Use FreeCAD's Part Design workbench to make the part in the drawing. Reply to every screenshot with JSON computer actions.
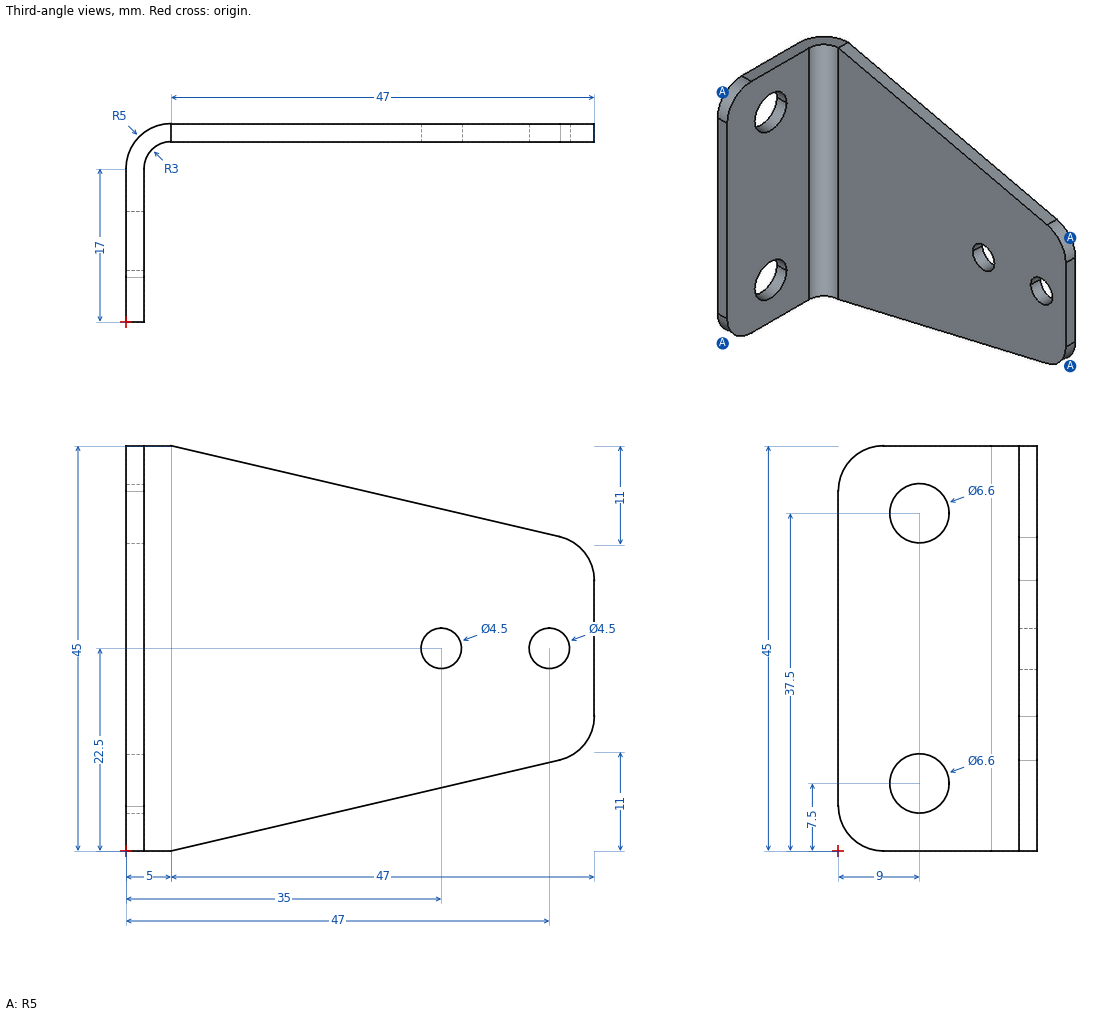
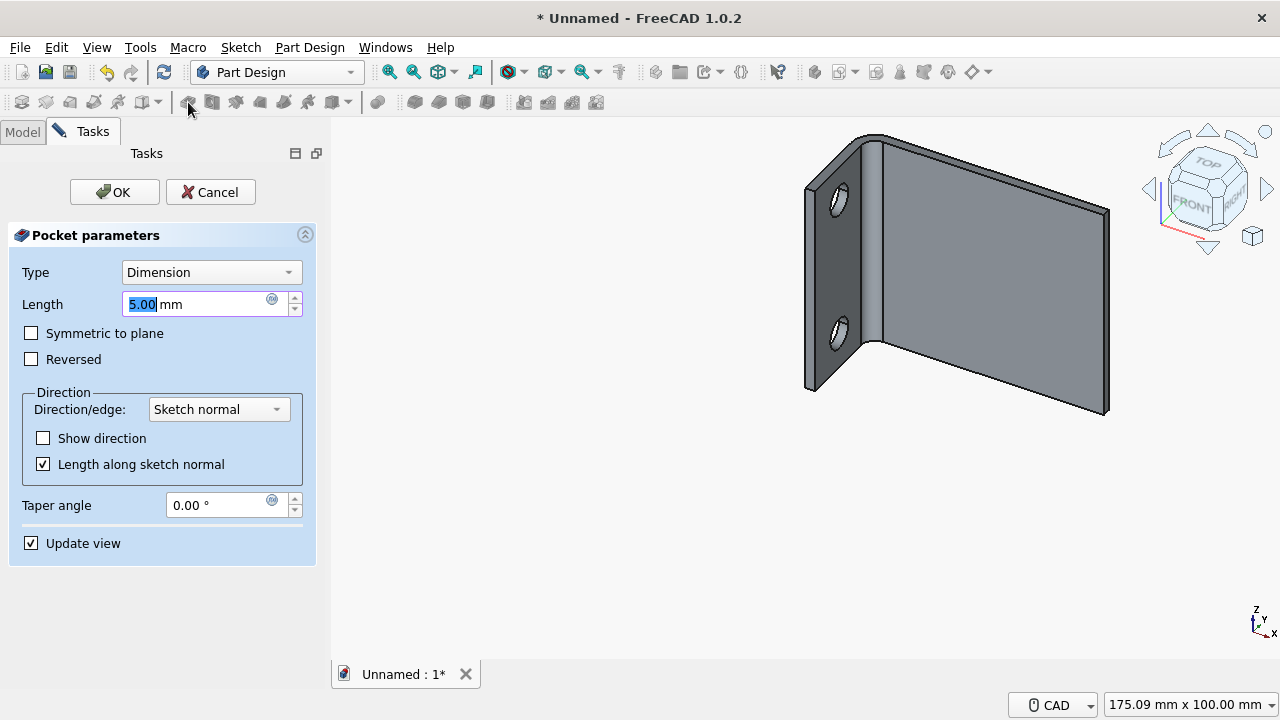
{"action": "left_click", "coordinate": [212, 272]}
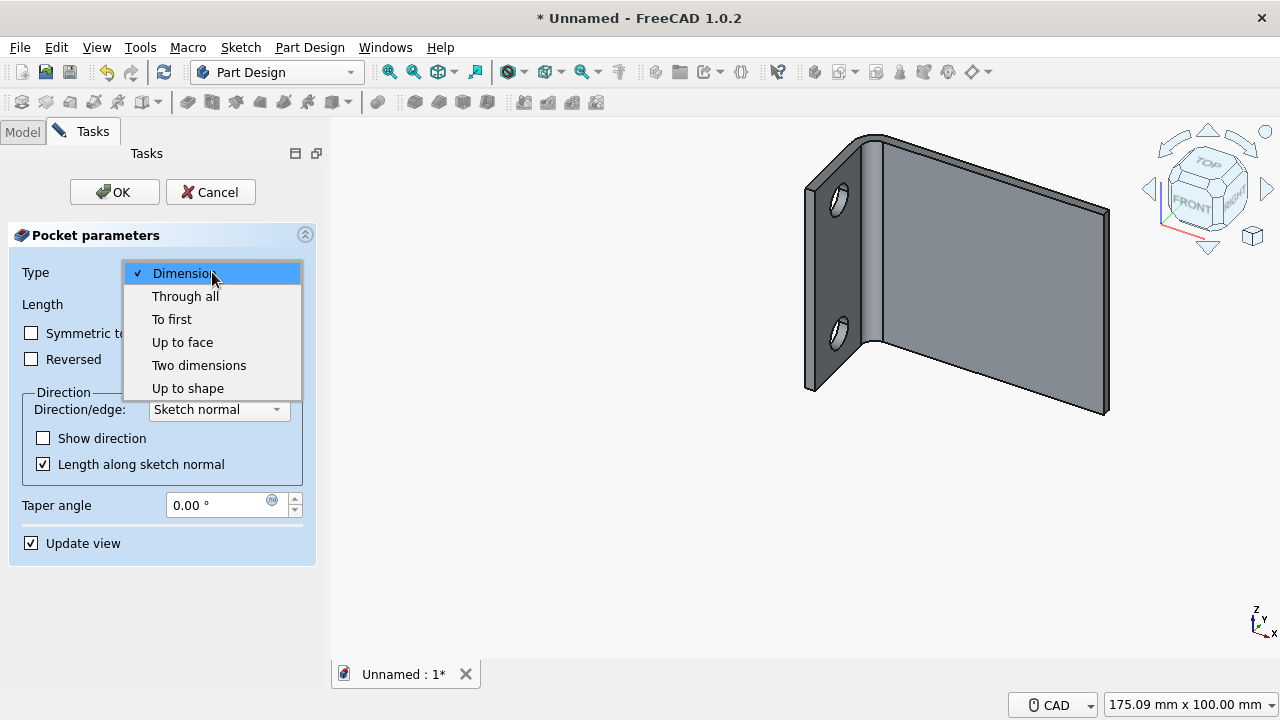
{"action": "left_click", "coordinate": [212, 320]}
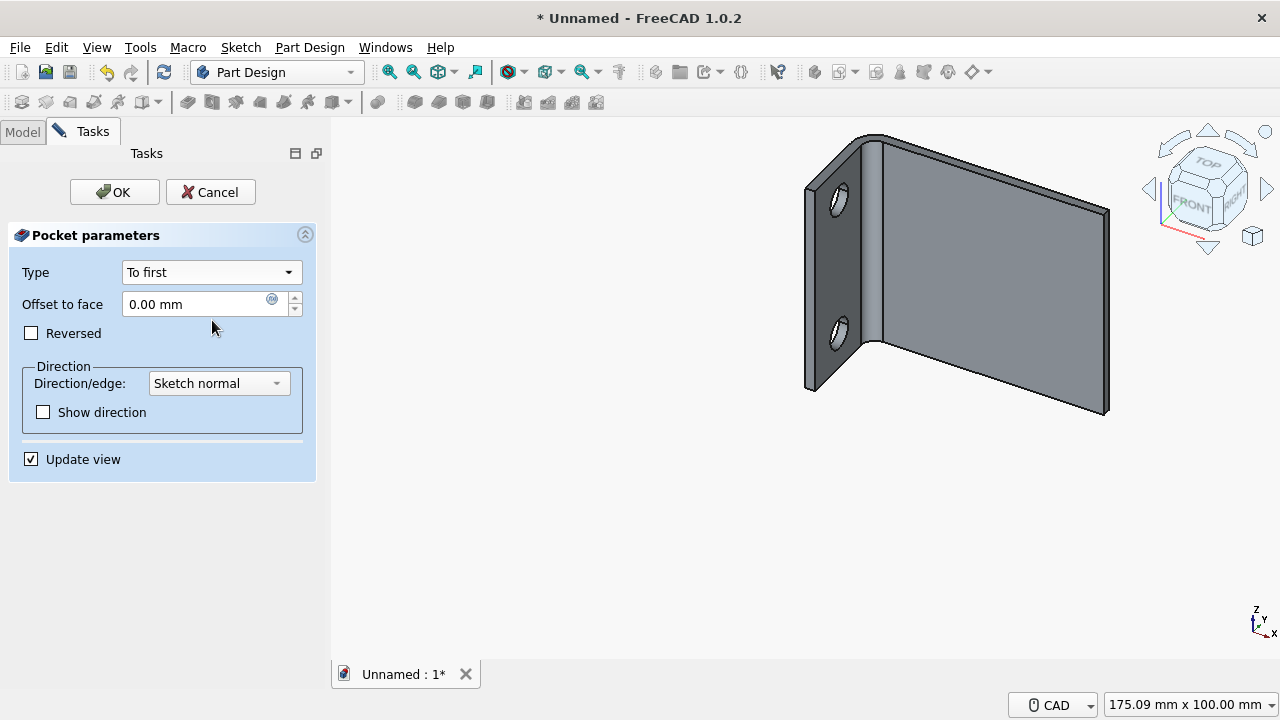
{"action": "left_click", "coordinate": [115, 192]}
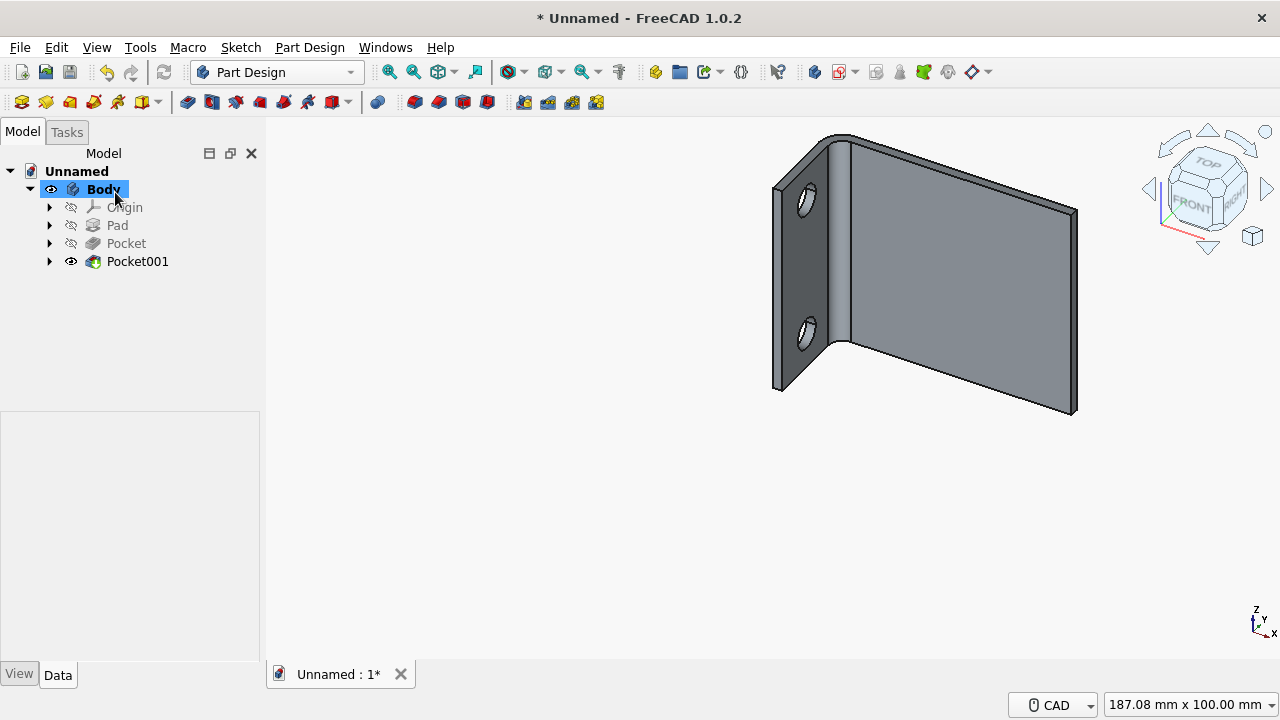
{"action": "key", "text": "4"}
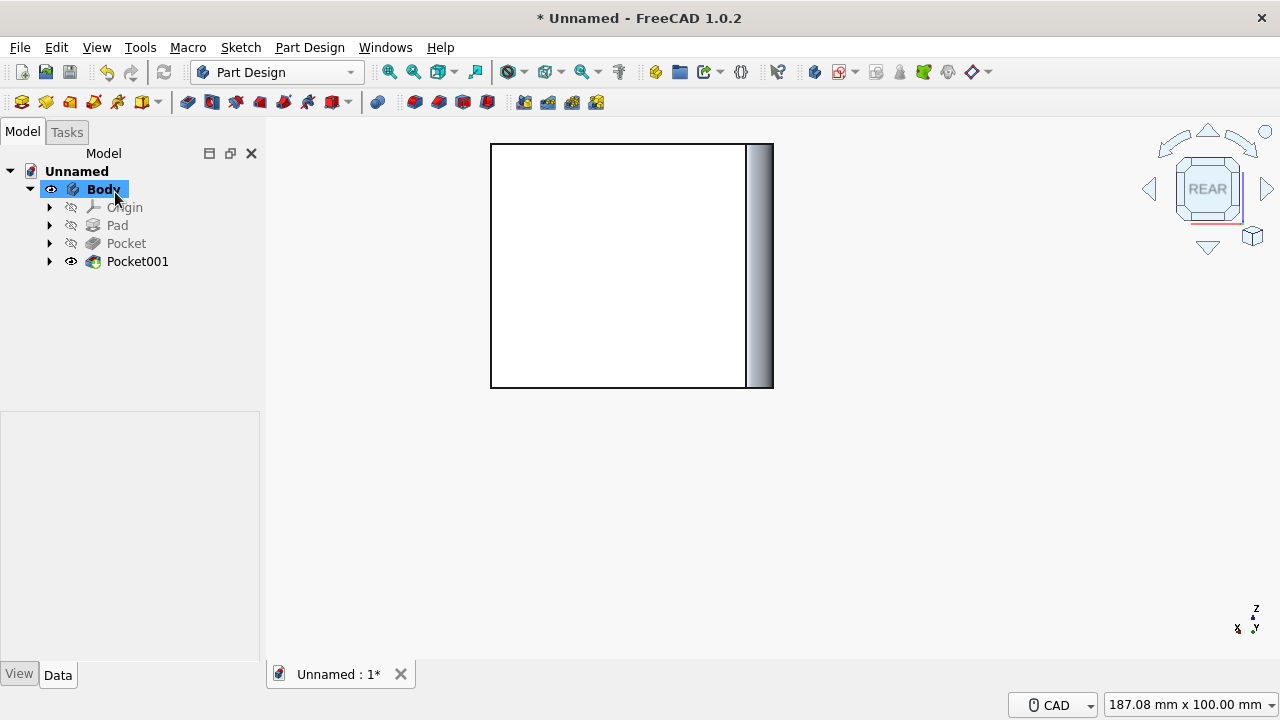
{"action": "left_click", "coordinate": [619, 265]}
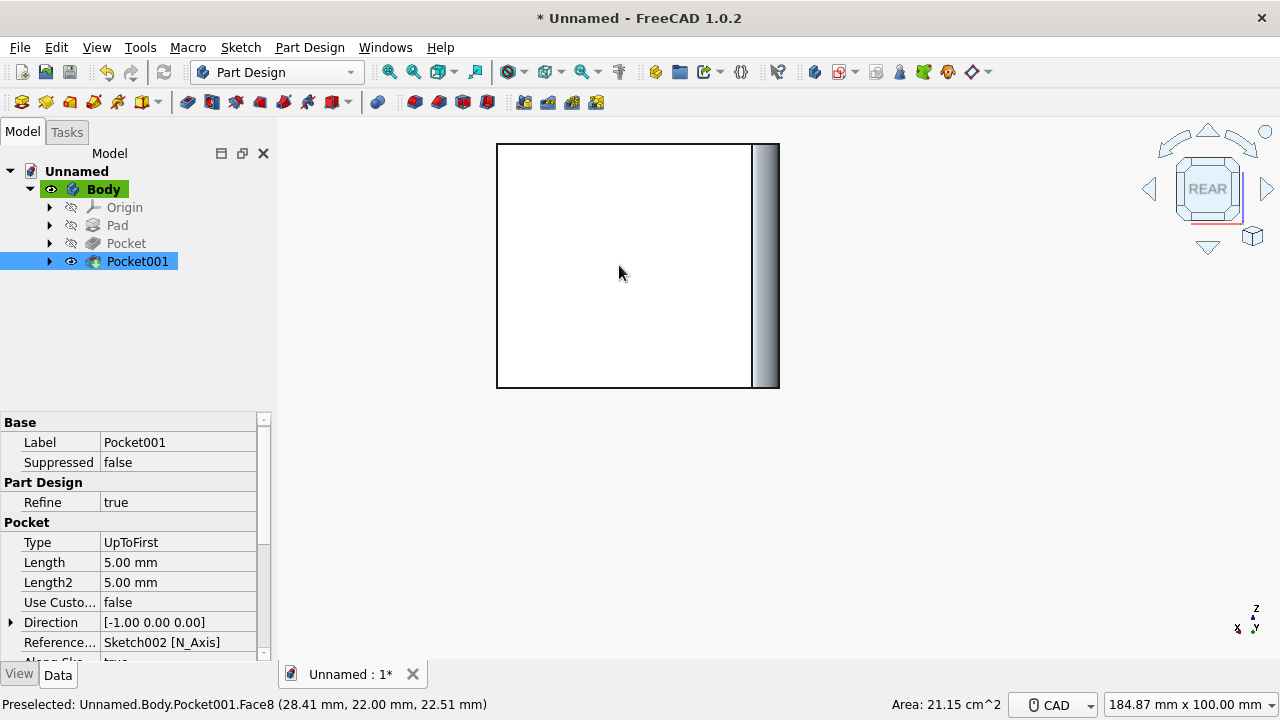
{"action": "left_click", "coordinate": [840, 72]}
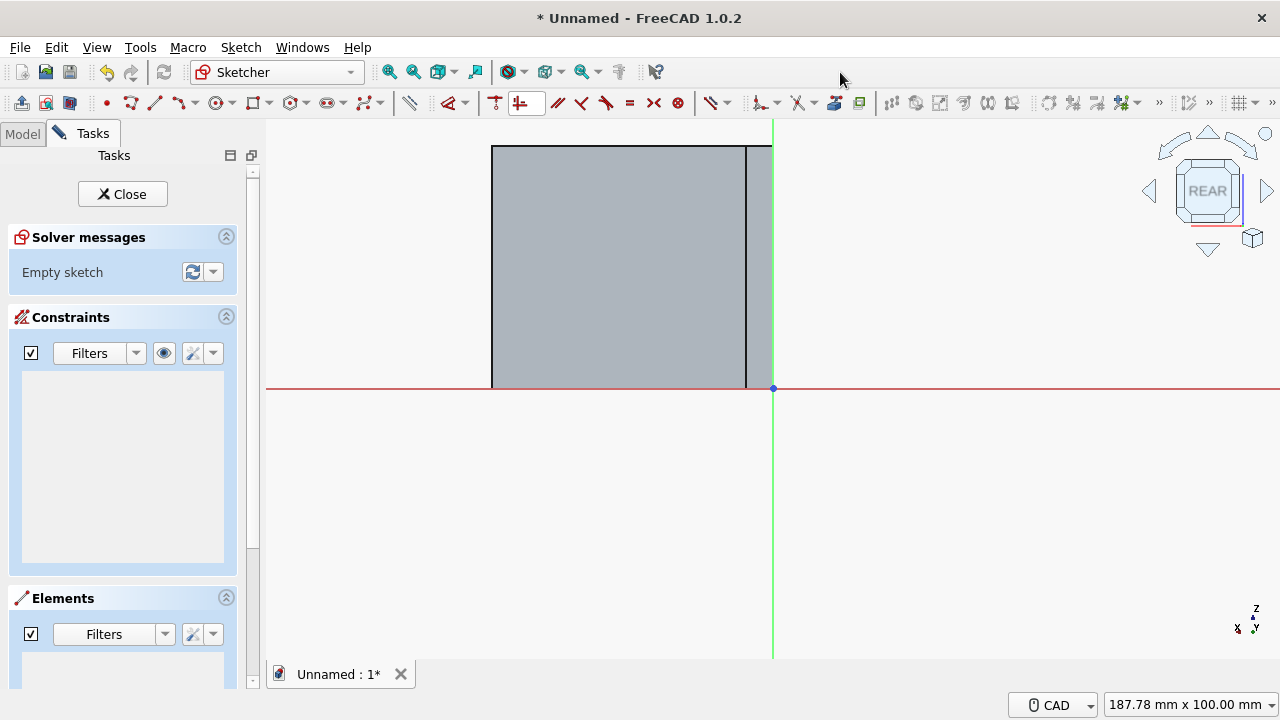
{"action": "scroll", "coordinate": [574, 258], "scroll_direction": "up", "scroll_amount": 13}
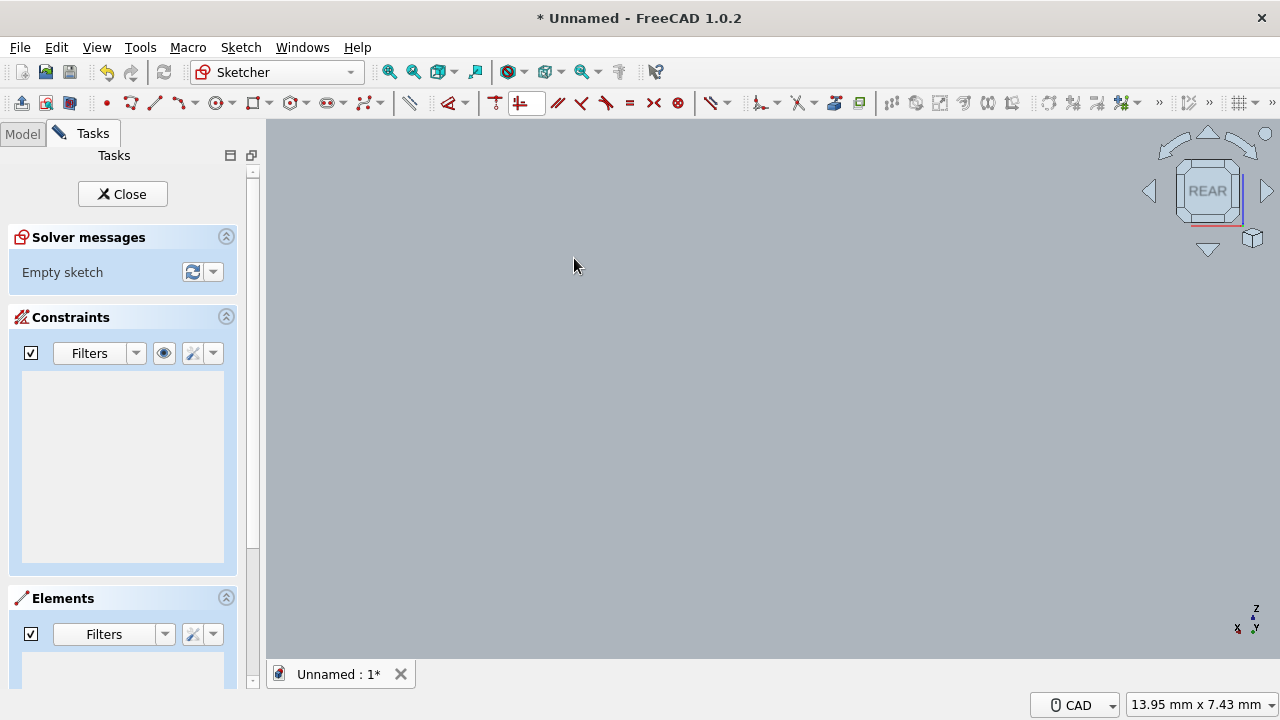
{"action": "key", "text": "g c"}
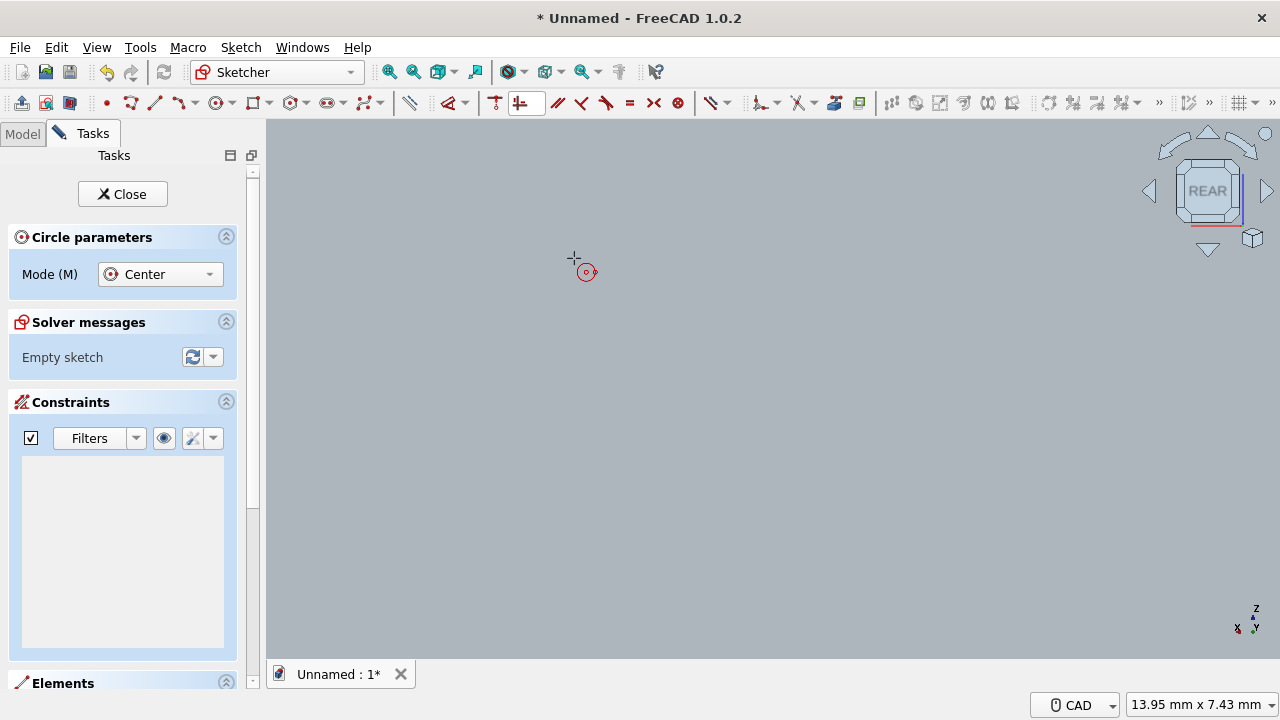
{"action": "left_click", "coordinate": [705, 383]}
{"action": "mouse_move", "coordinate": [821, 267]}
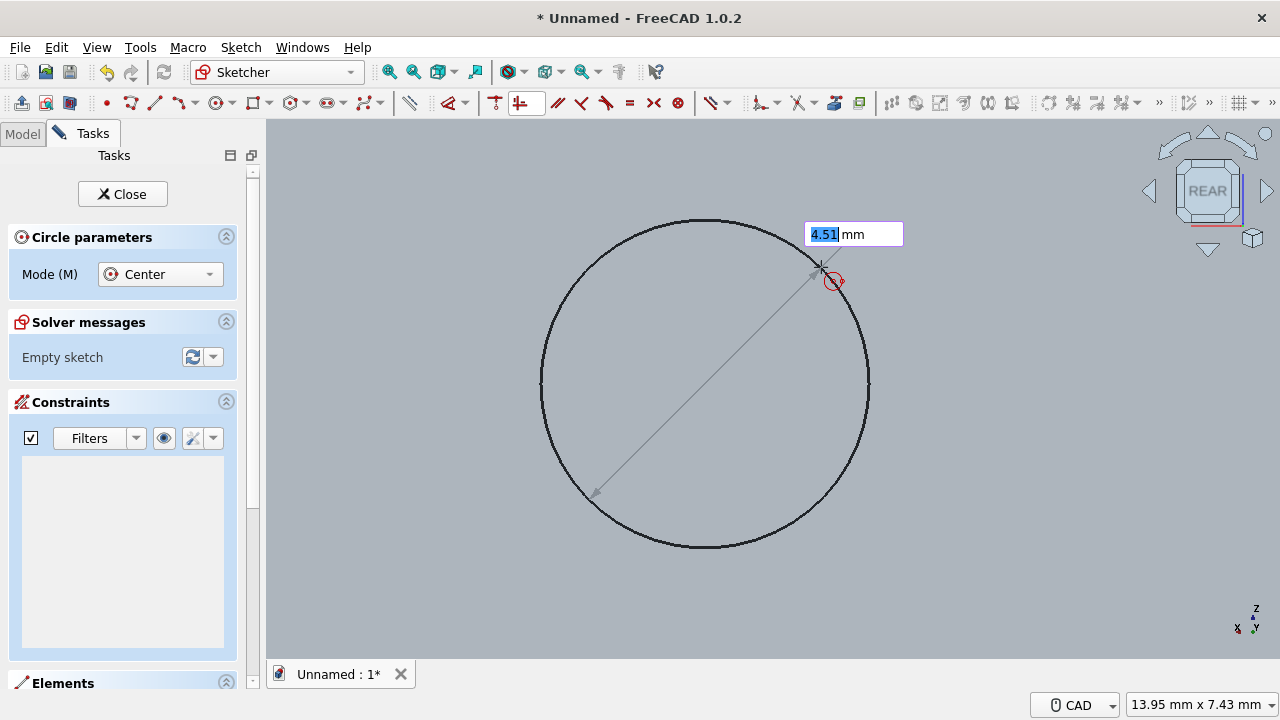
{"action": "type", "text": "4.5"}
{"action": "key", "text": "Return"}
{"action": "key", "text": "Escape"}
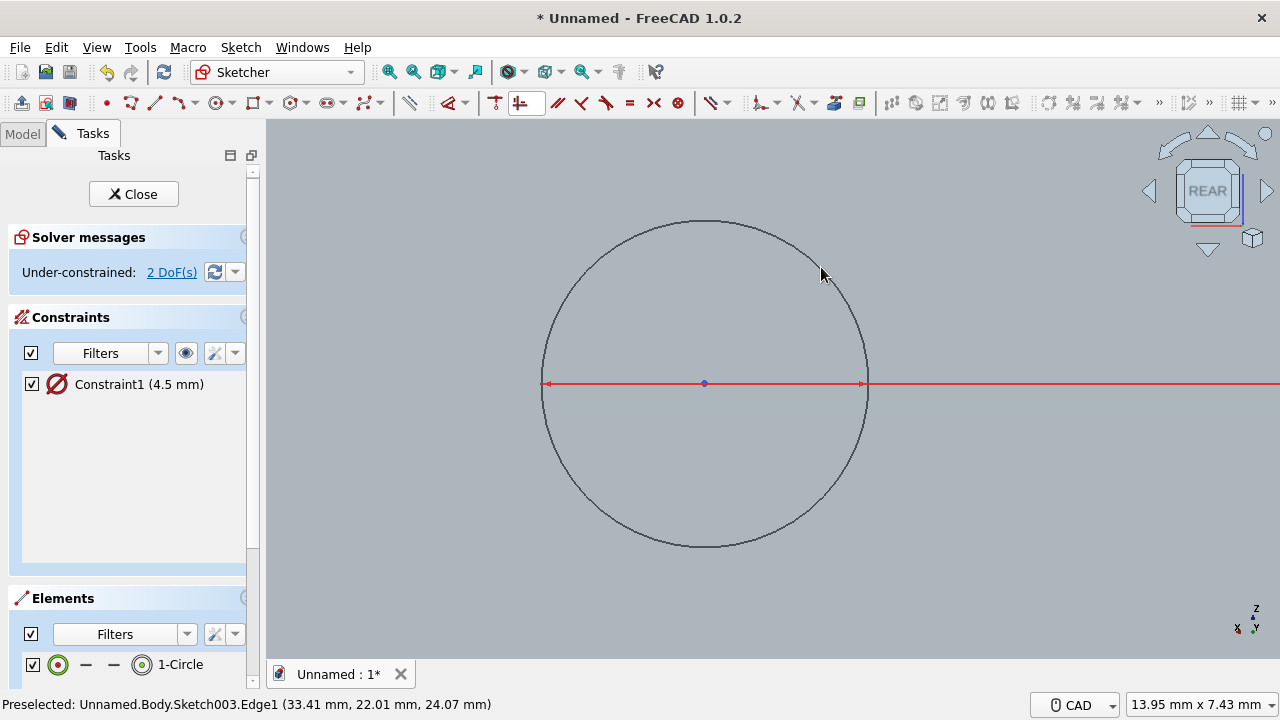
{"action": "key", "text": "d"}